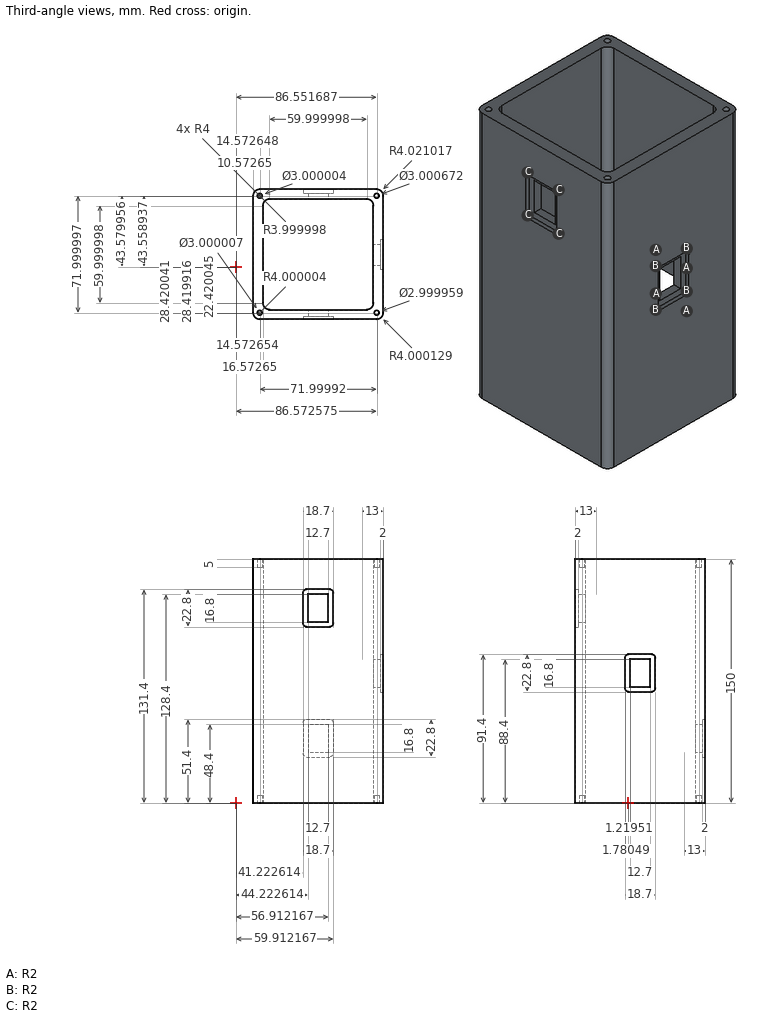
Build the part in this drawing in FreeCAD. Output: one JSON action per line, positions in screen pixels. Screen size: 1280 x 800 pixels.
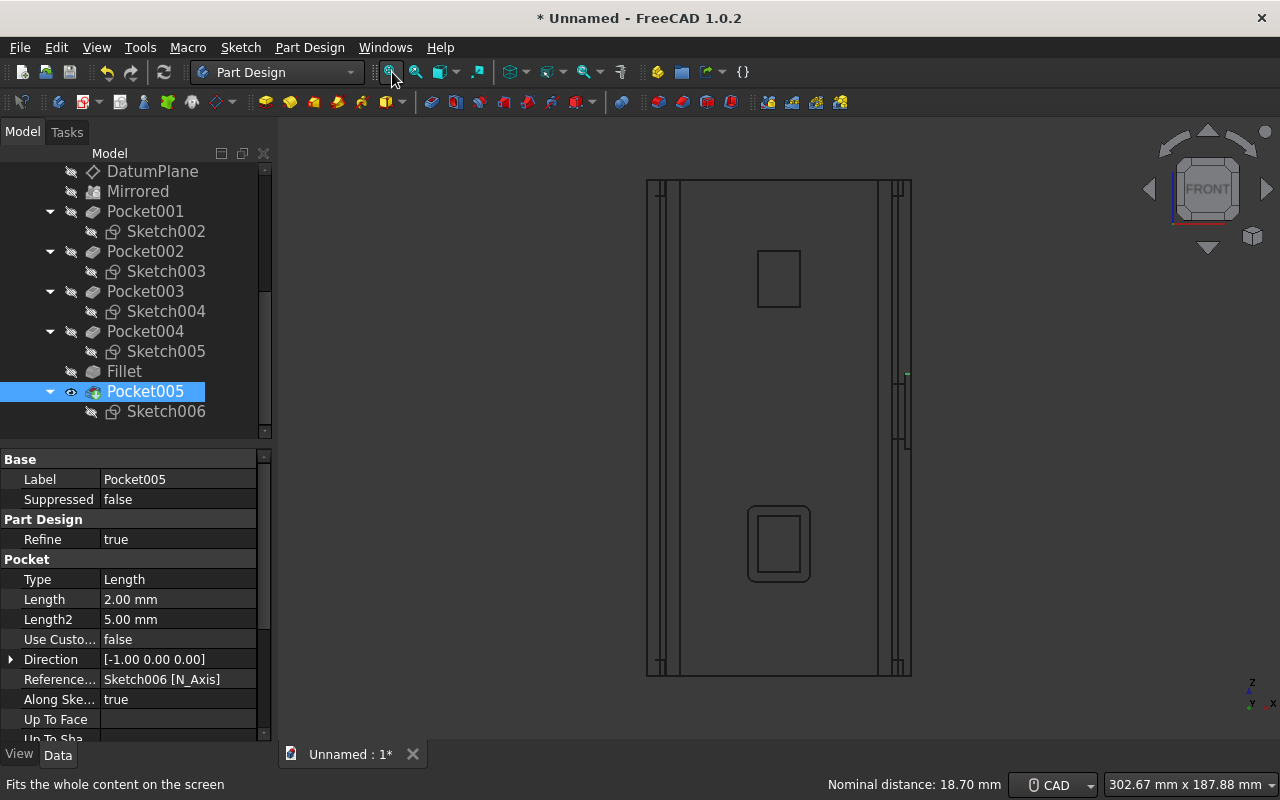
{"action": "scroll", "coordinate": [908, 448], "scroll_direction": "up", "scroll_amount": 9}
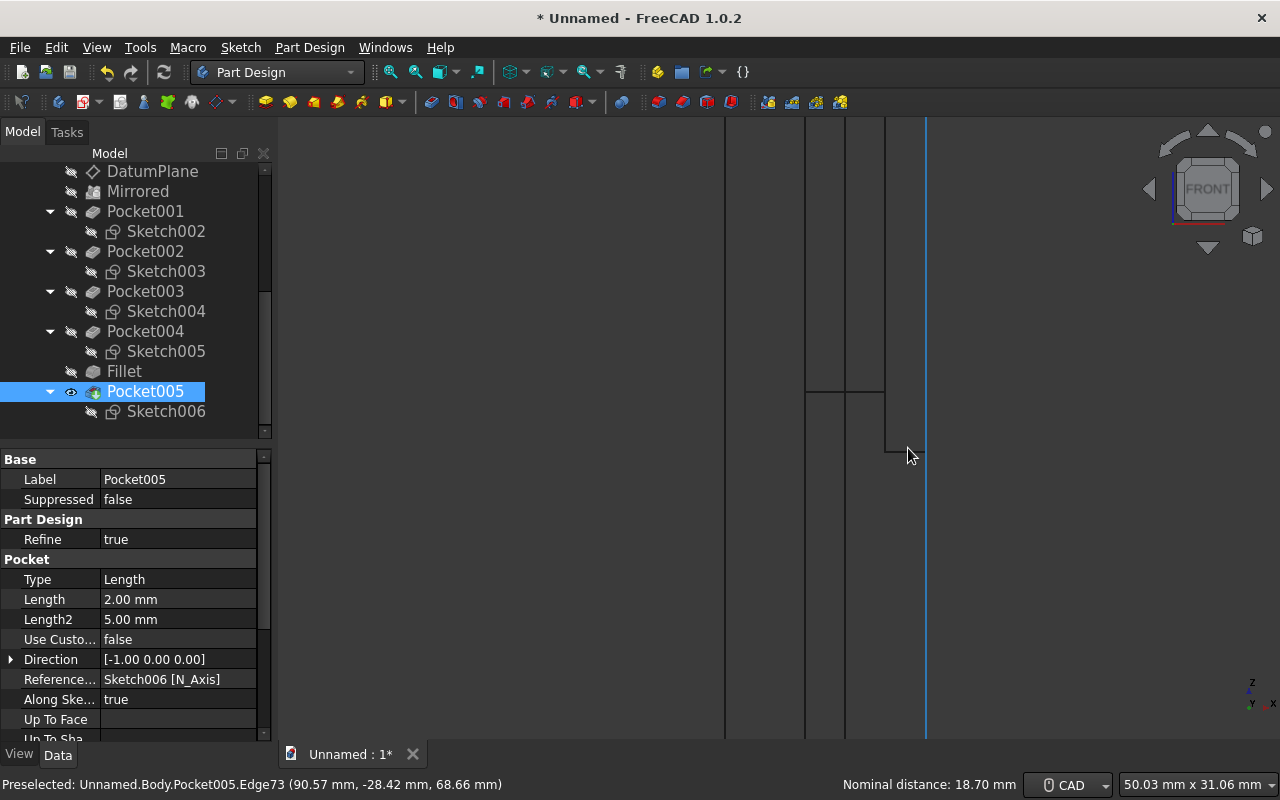
{"action": "left_click", "coordinate": [906, 451], "text": "ctrl"}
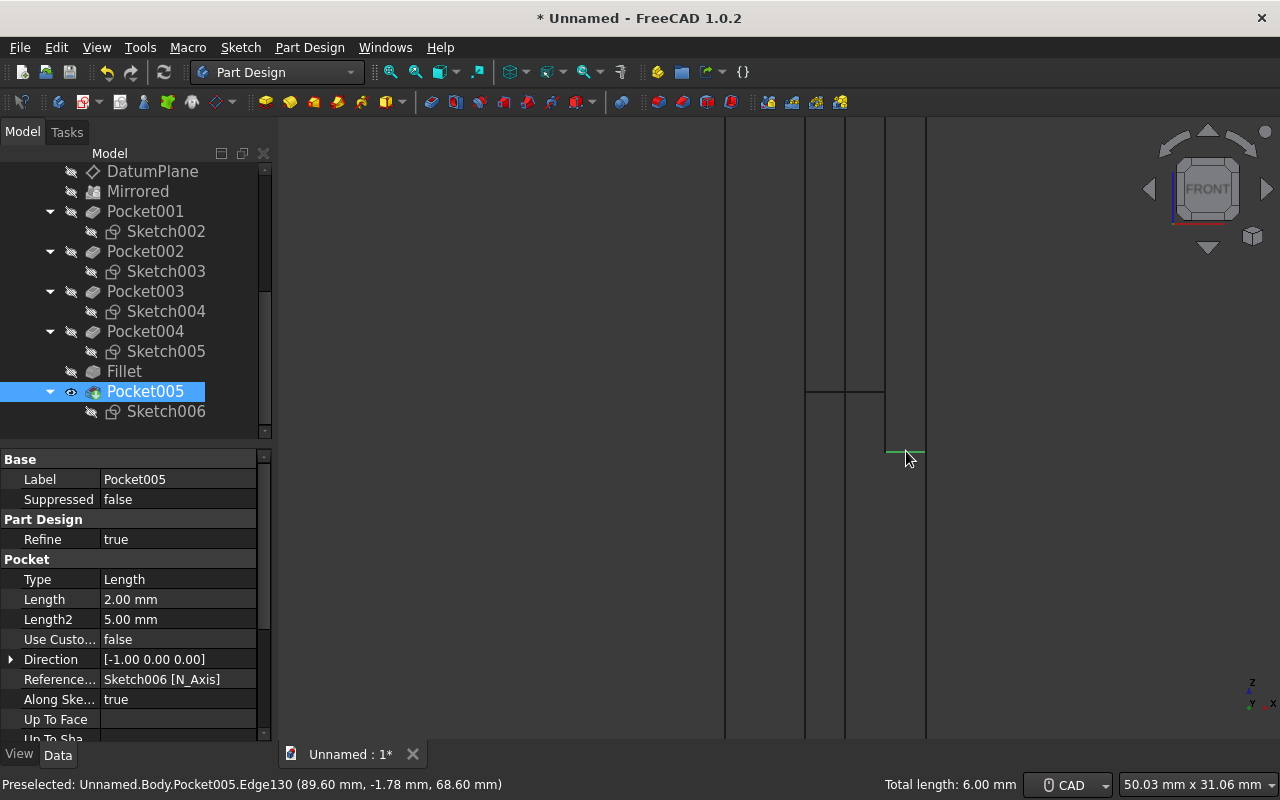
{"action": "left_click", "coordinate": [392, 72]}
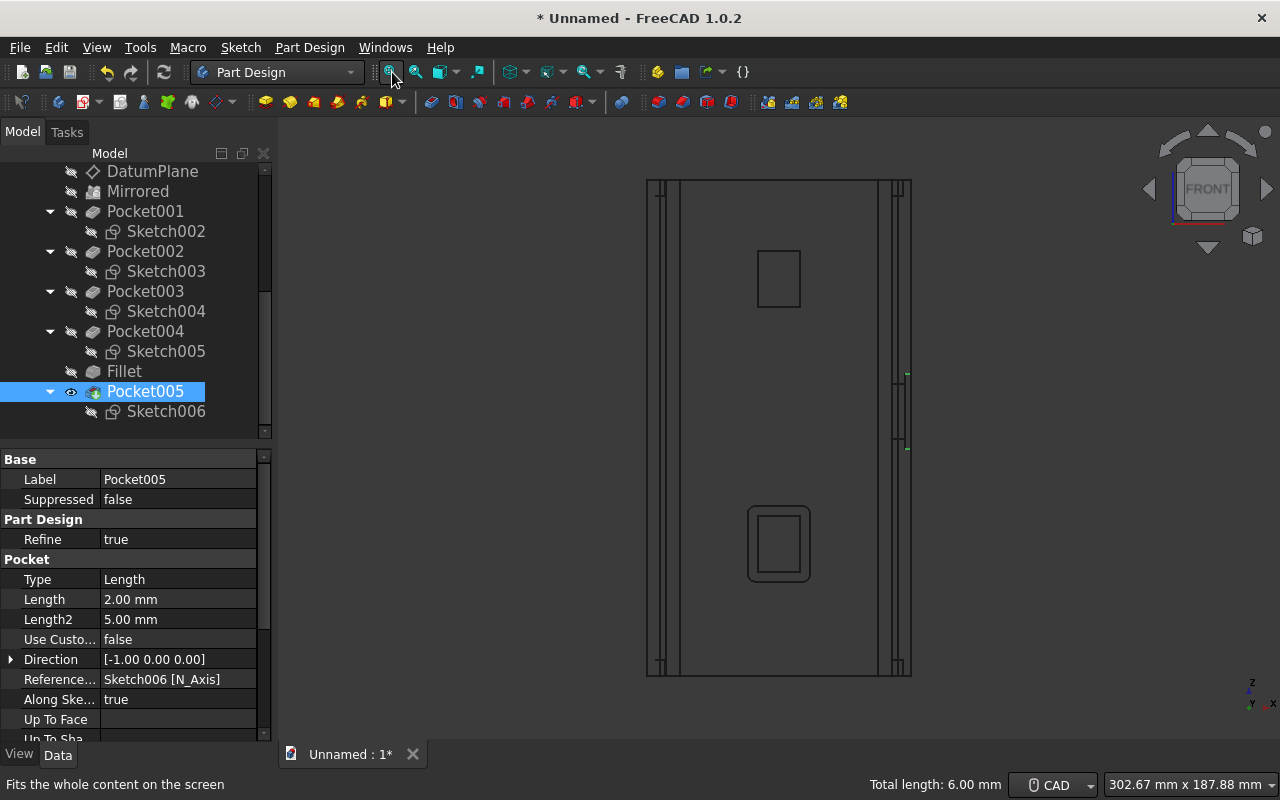
{"action": "key", "text": "3"}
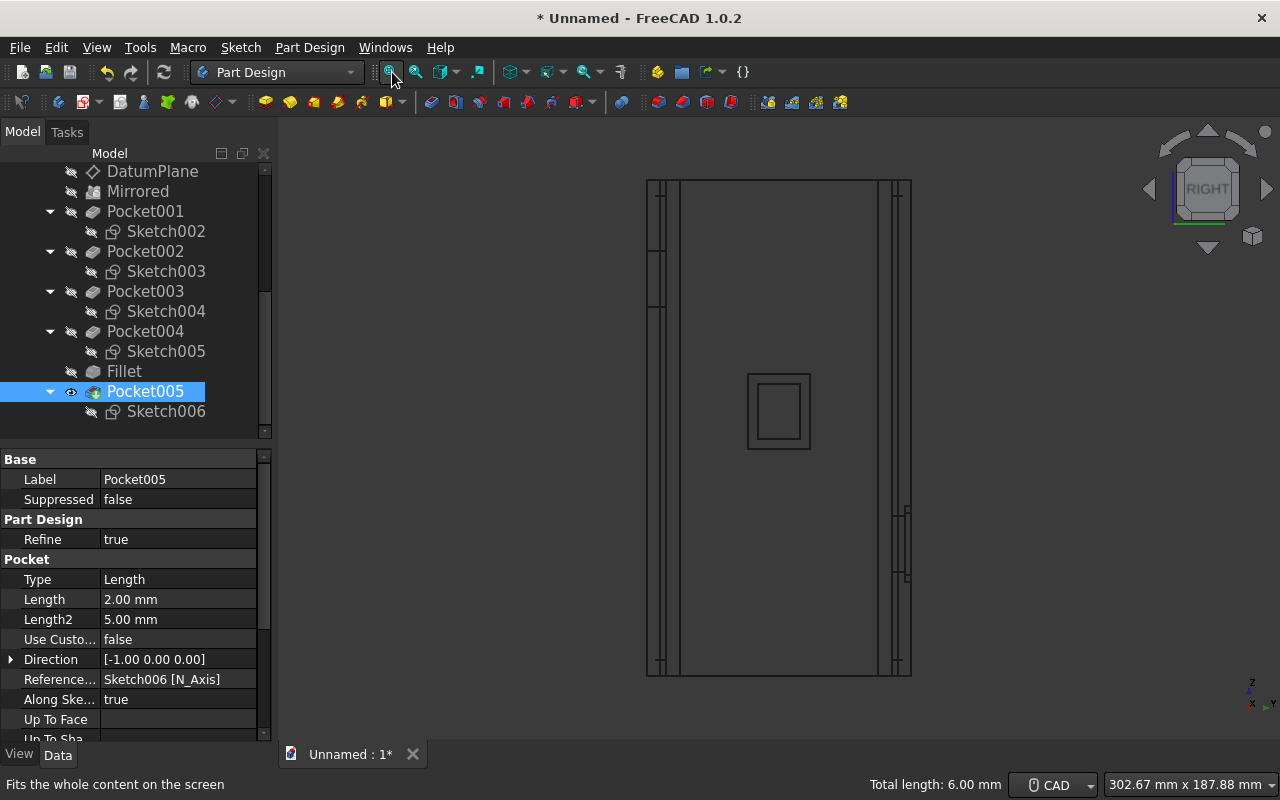
{"action": "scroll", "coordinate": [810, 448], "scroll_direction": "up", "scroll_amount": 9}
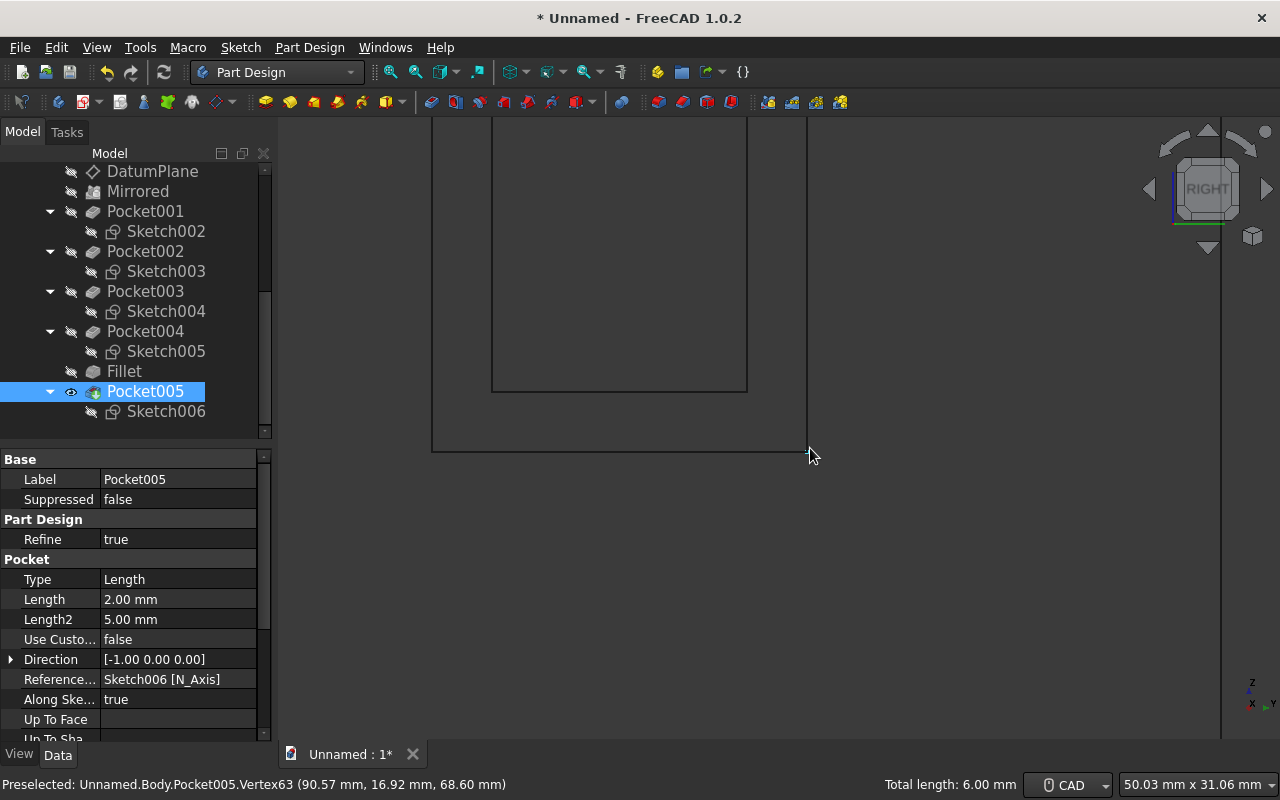
{"action": "left_click", "coordinate": [392, 72]}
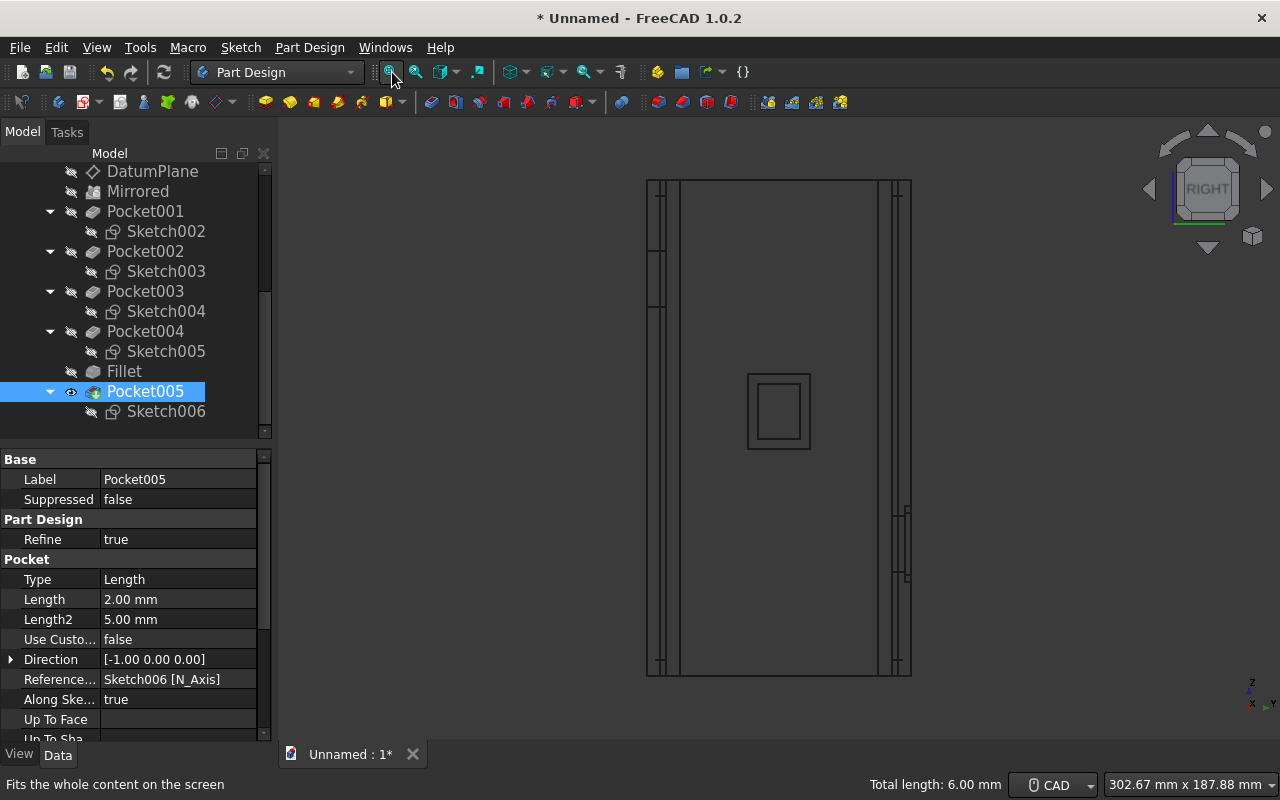
{"action": "key", "text": "5"}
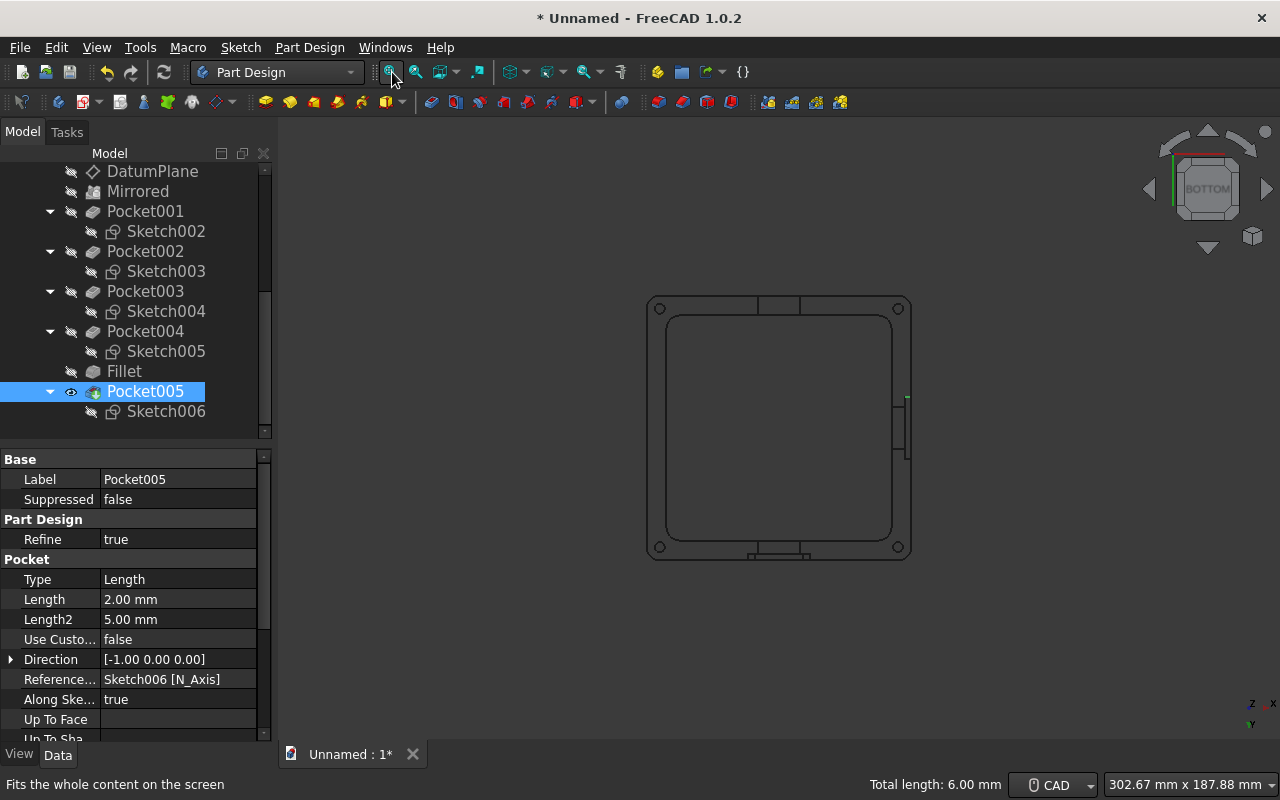
{"action": "left_click", "coordinate": [392, 72]}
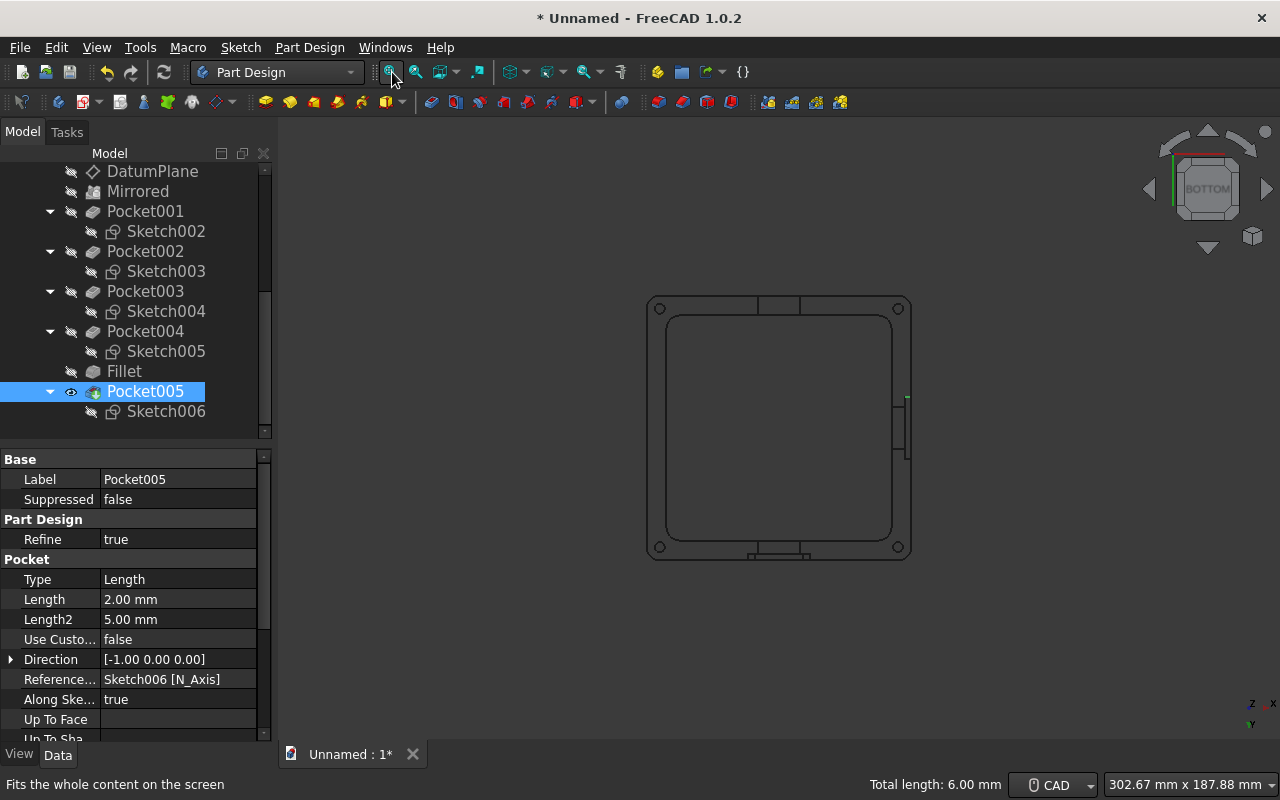
{"action": "scroll", "coordinate": [908, 458], "scroll_direction": "up", "scroll_amount": 9}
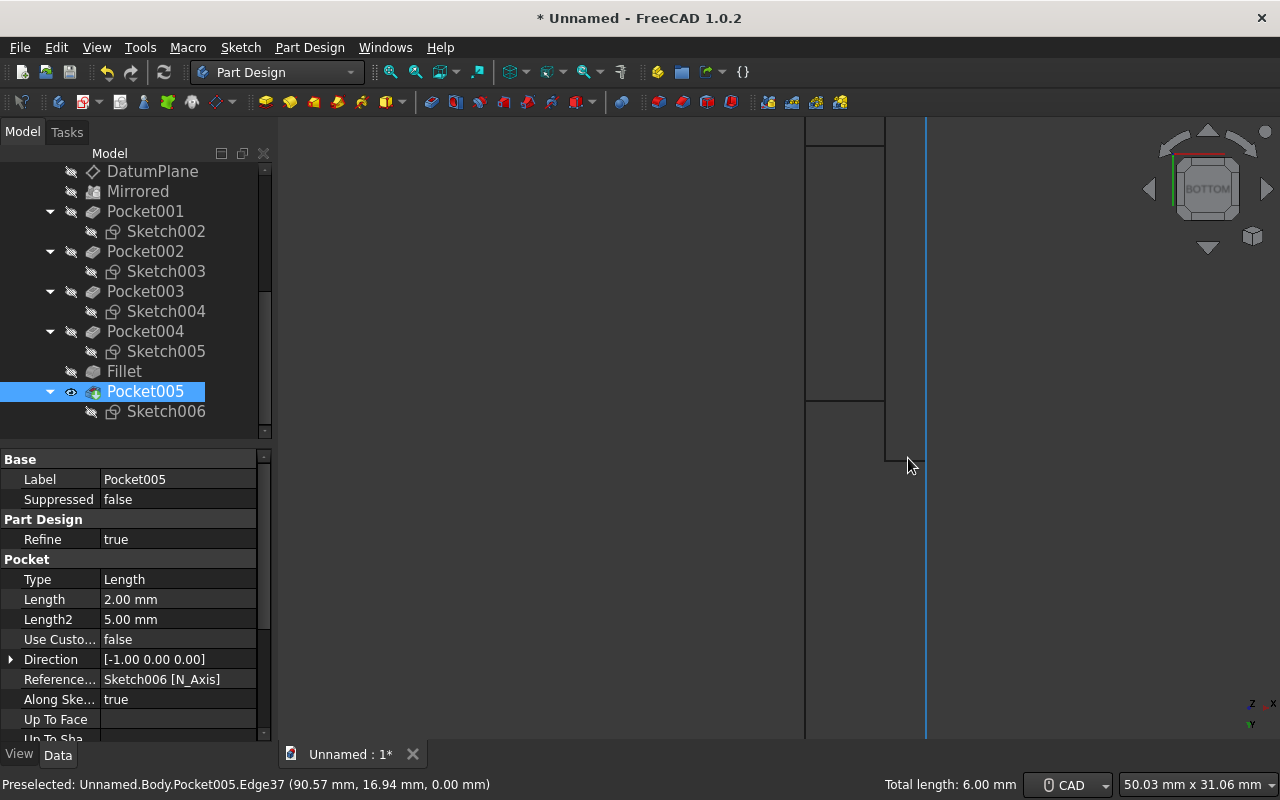
{"action": "left_click", "coordinate": [906, 460], "text": "ctrl"}